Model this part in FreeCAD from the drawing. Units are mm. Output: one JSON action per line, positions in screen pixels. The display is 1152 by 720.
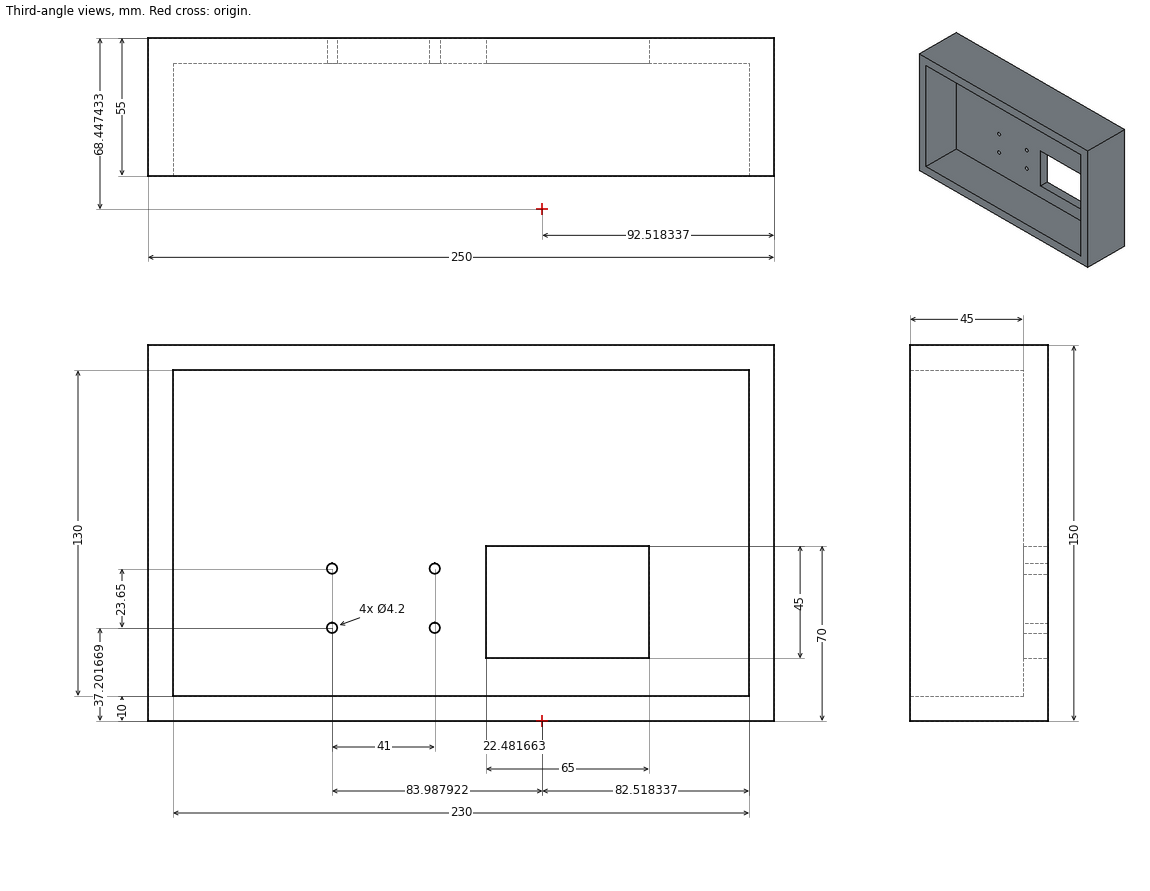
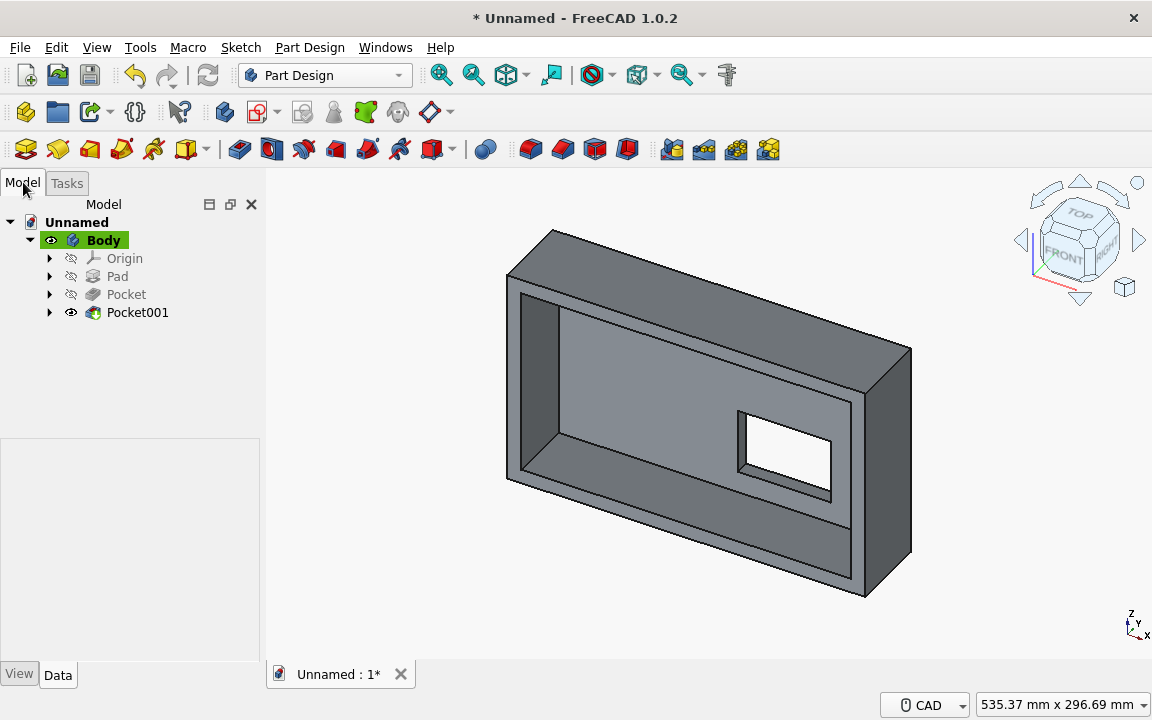
{"action": "left_click", "coordinate": [50, 258]}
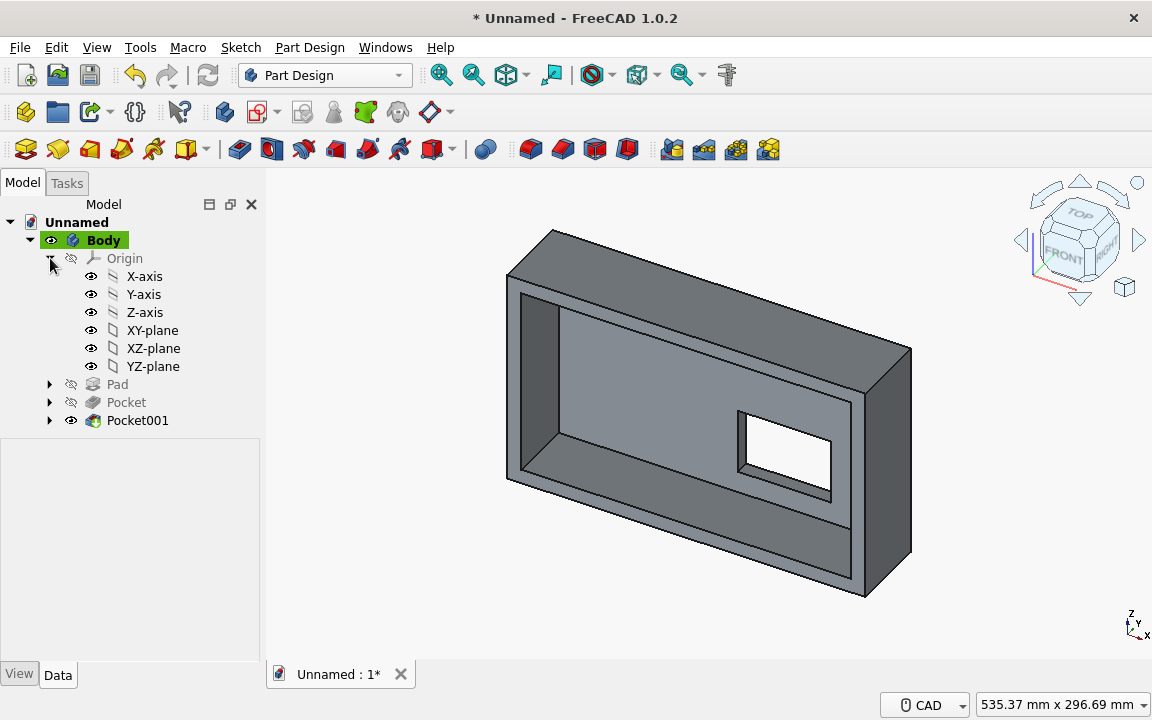
{"action": "left_click", "coordinate": [136, 348]}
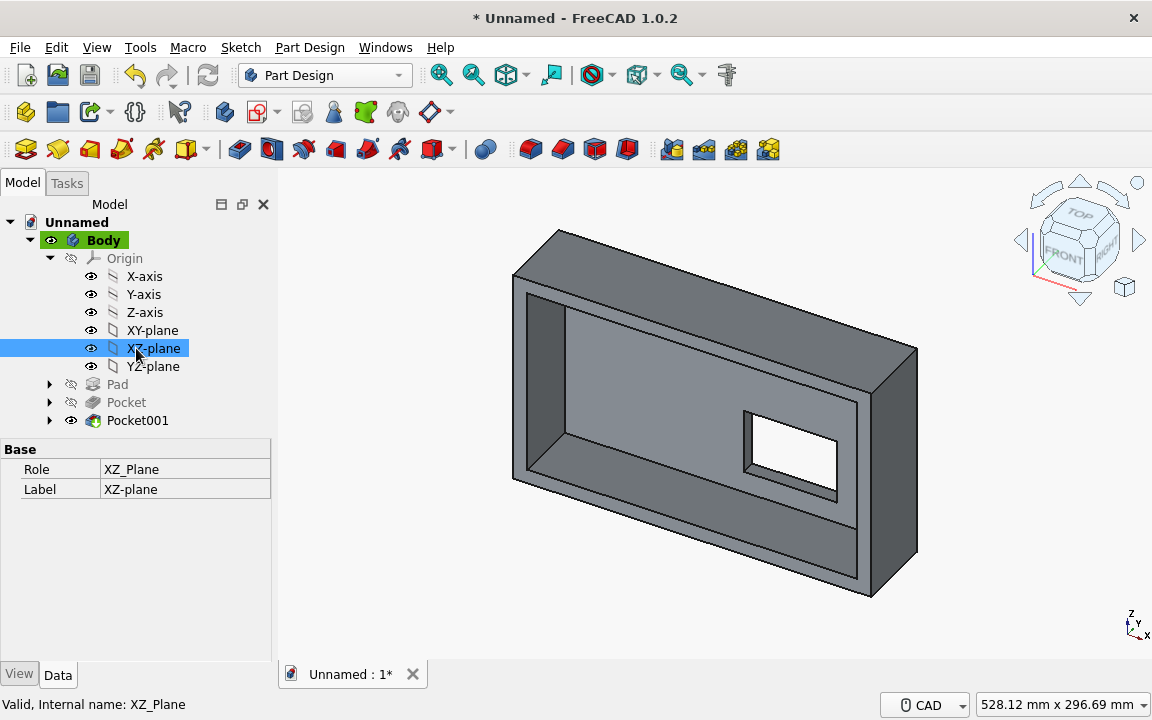
{"action": "left_click", "coordinate": [430, 112]}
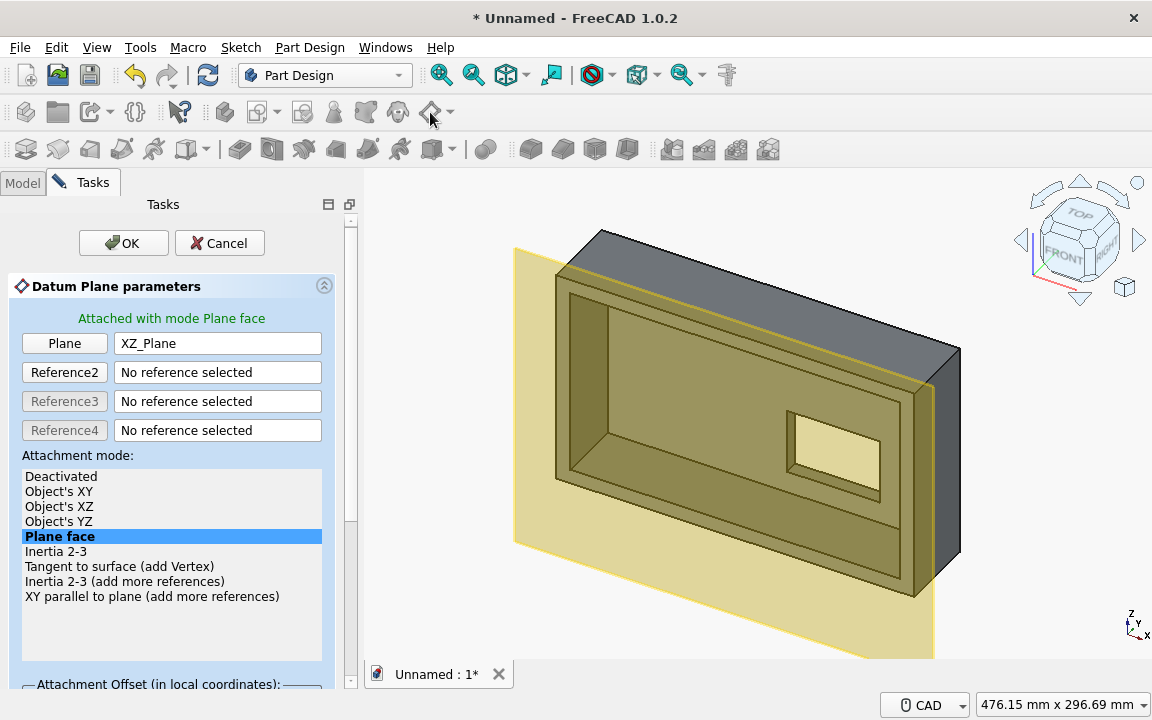
{"action": "scroll", "coordinate": [351, 451], "scroll_direction": "down", "scroll_amount": 3}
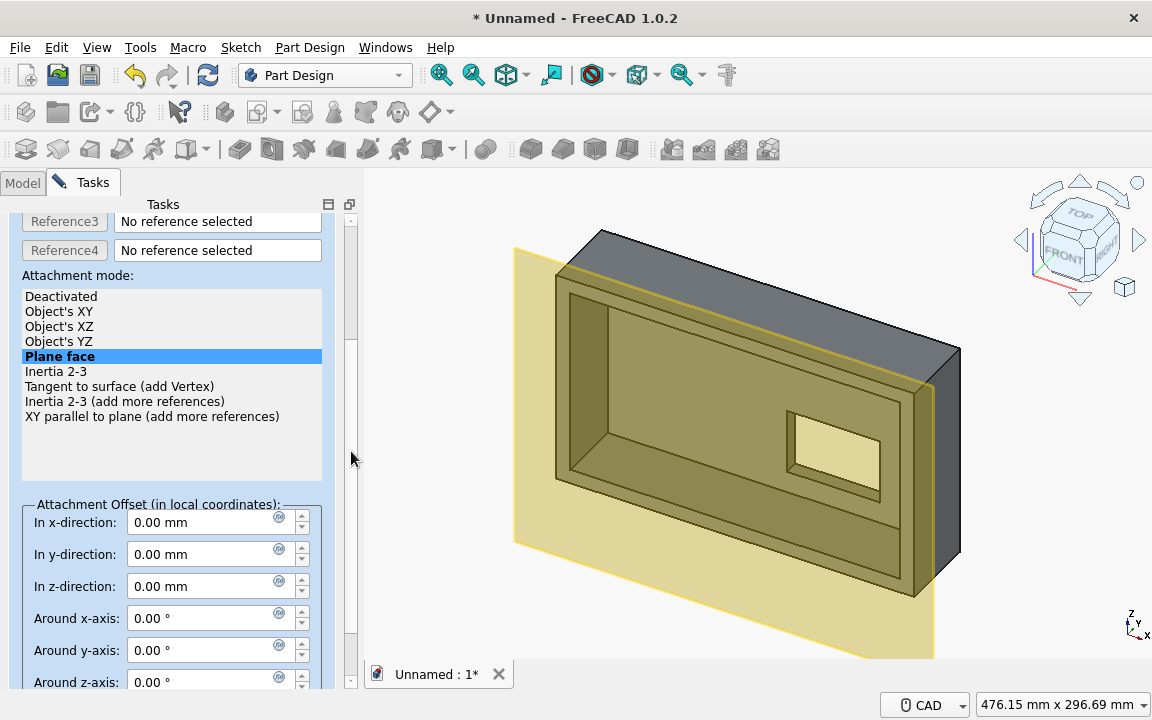
{"action": "triple_click", "coordinate": [210, 586]}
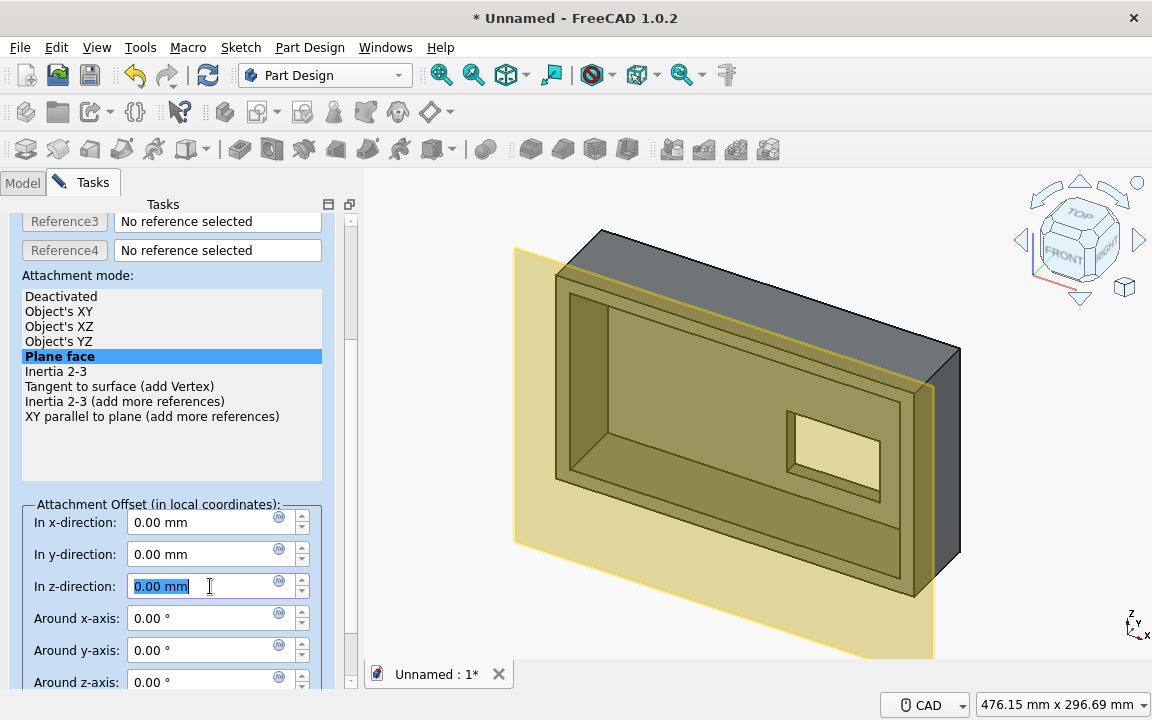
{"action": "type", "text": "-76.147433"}
{"action": "key", "text": "Tab"}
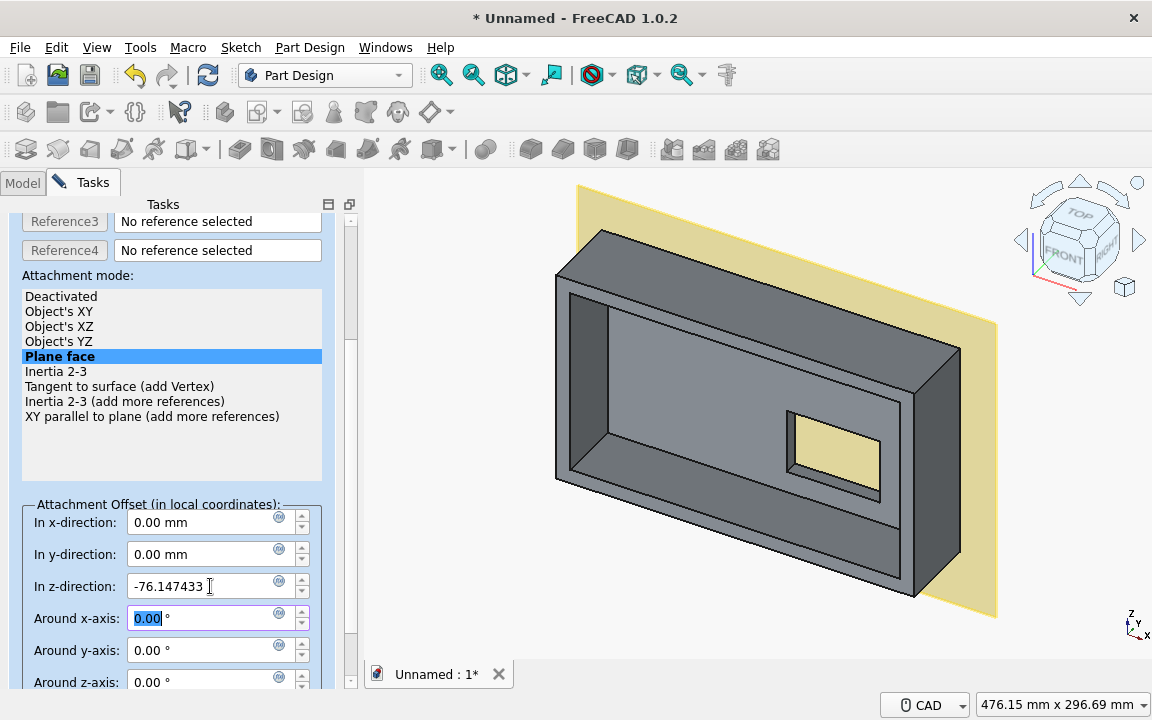
{"action": "scroll", "coordinate": [351, 451], "scroll_direction": "up", "scroll_amount": 4}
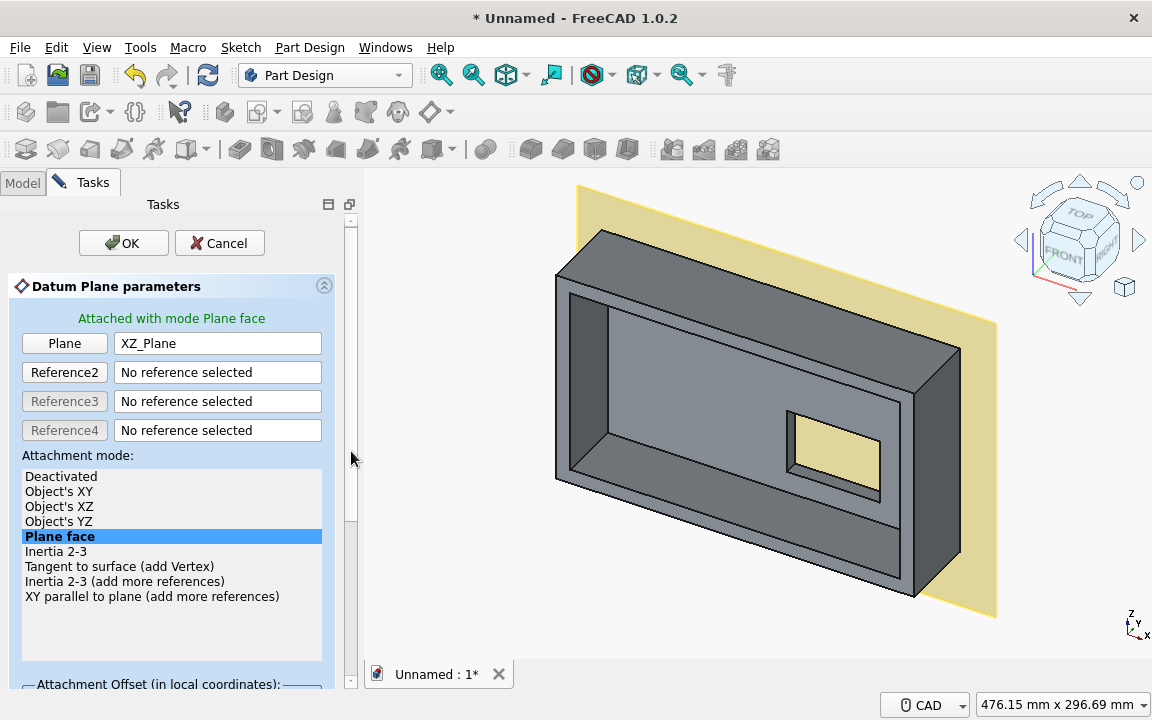
{"action": "left_click", "coordinate": [124, 243]}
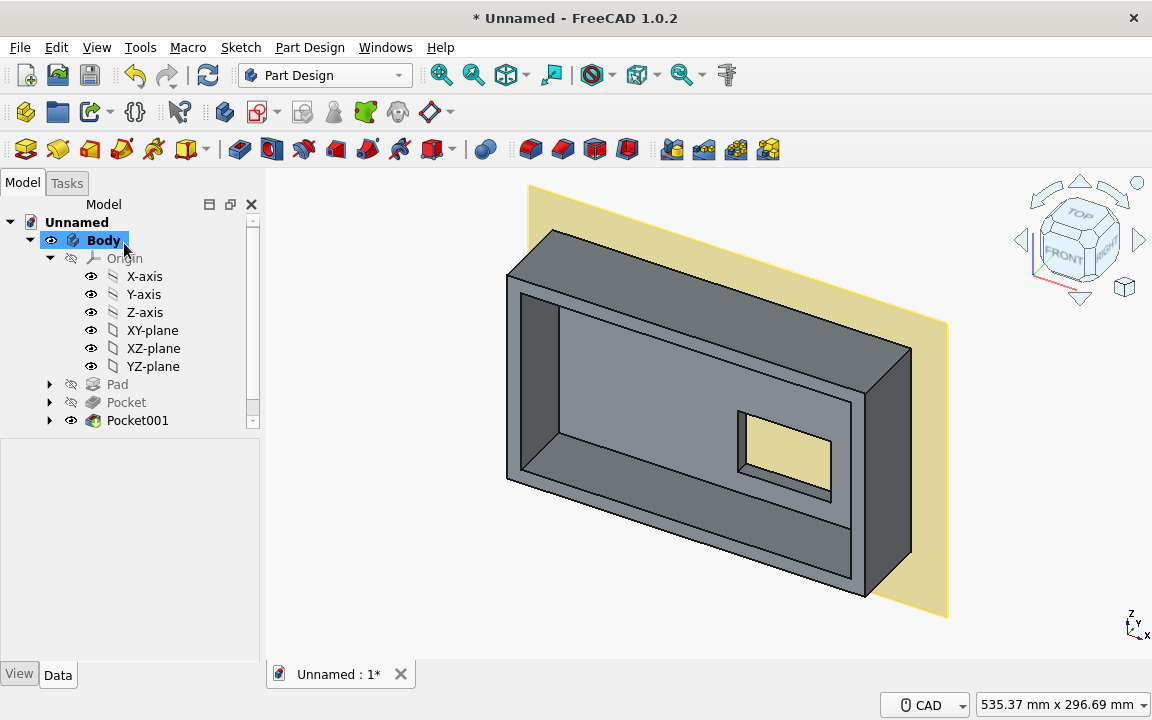
{"action": "scroll", "coordinate": [100, 326], "scroll_direction": "down", "scroll_amount": 3}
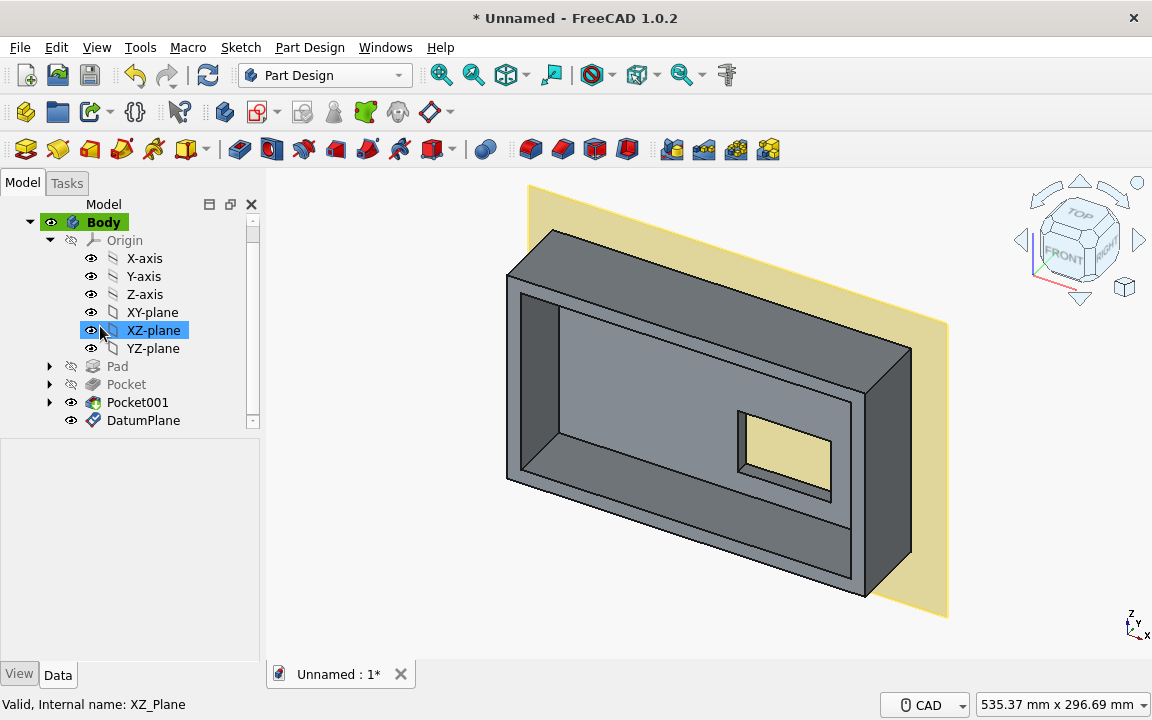
{"action": "left_click", "coordinate": [116, 420]}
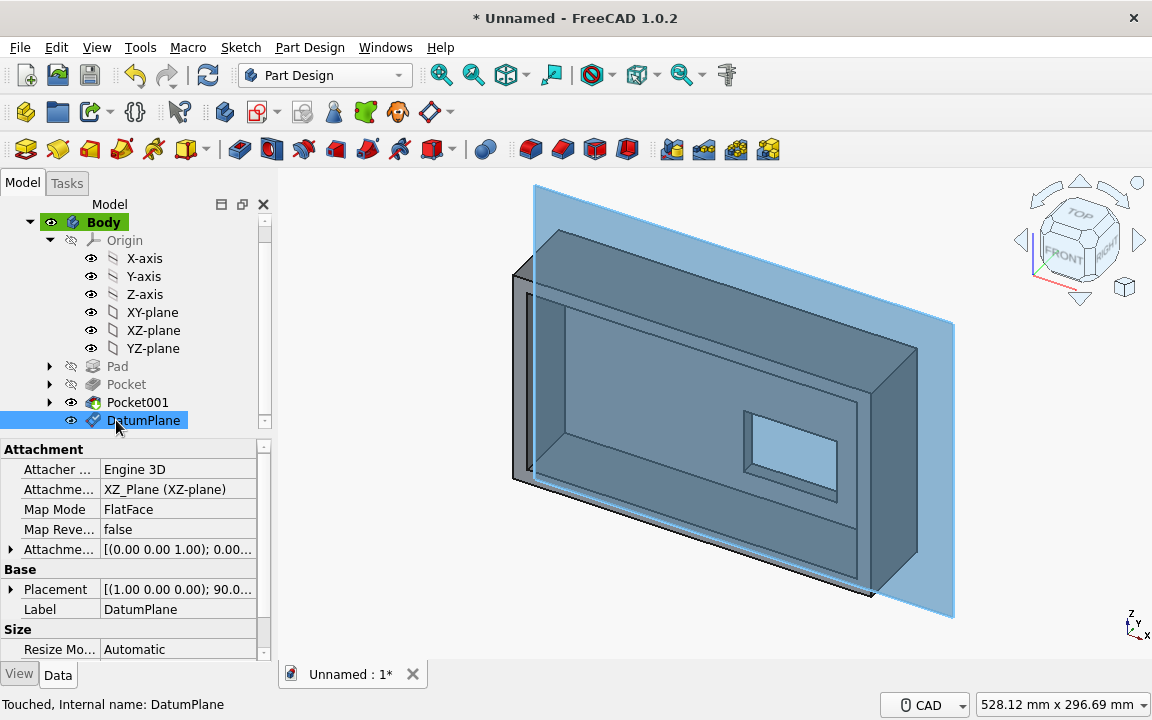
{"action": "left_click", "coordinate": [258, 112]}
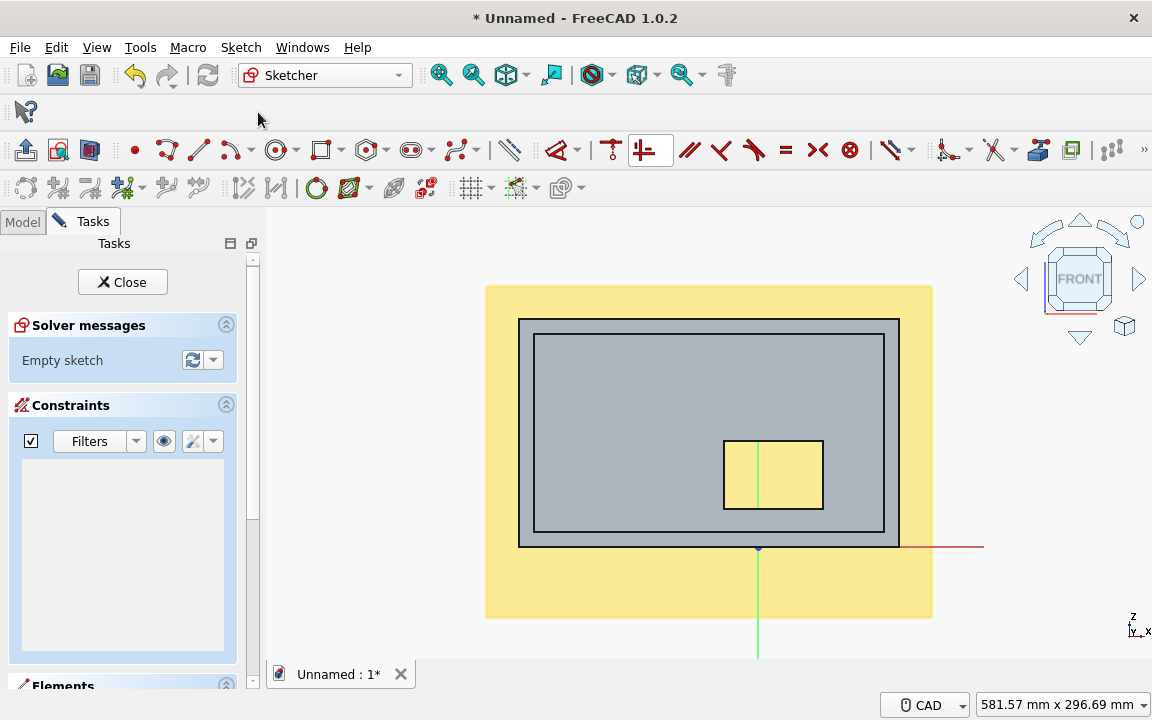
{"action": "left_click", "coordinate": [90, 150]}